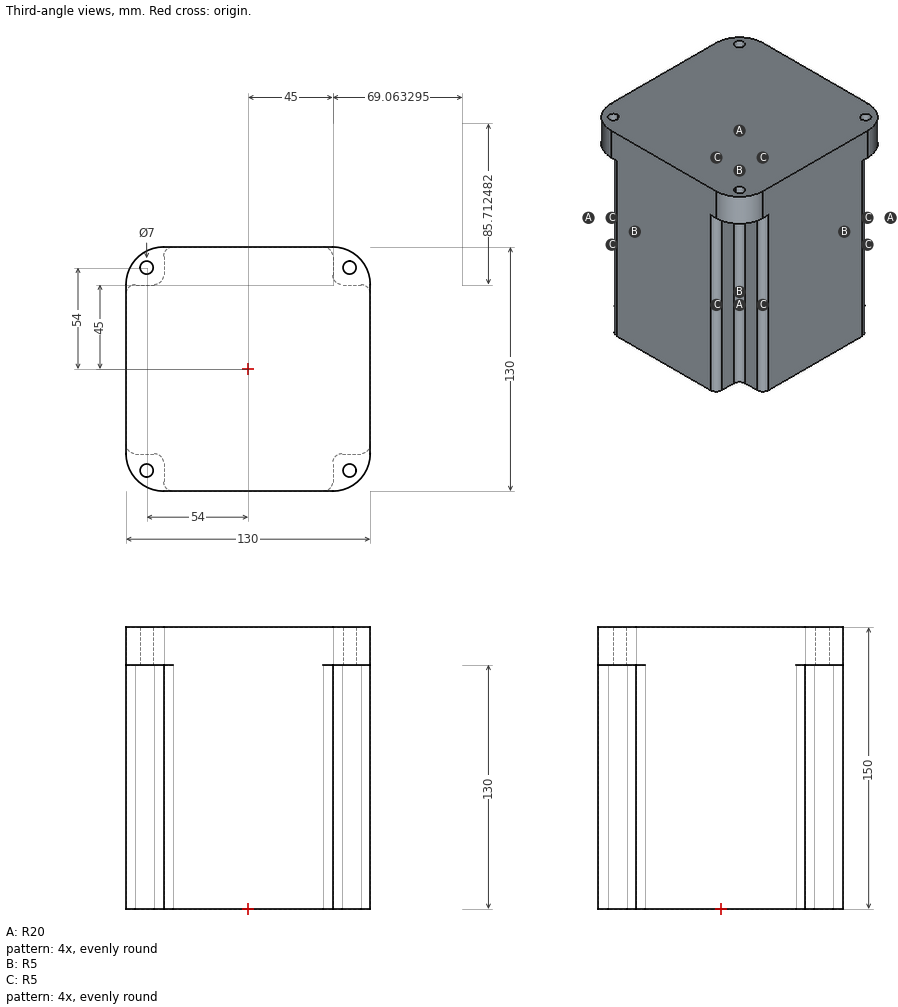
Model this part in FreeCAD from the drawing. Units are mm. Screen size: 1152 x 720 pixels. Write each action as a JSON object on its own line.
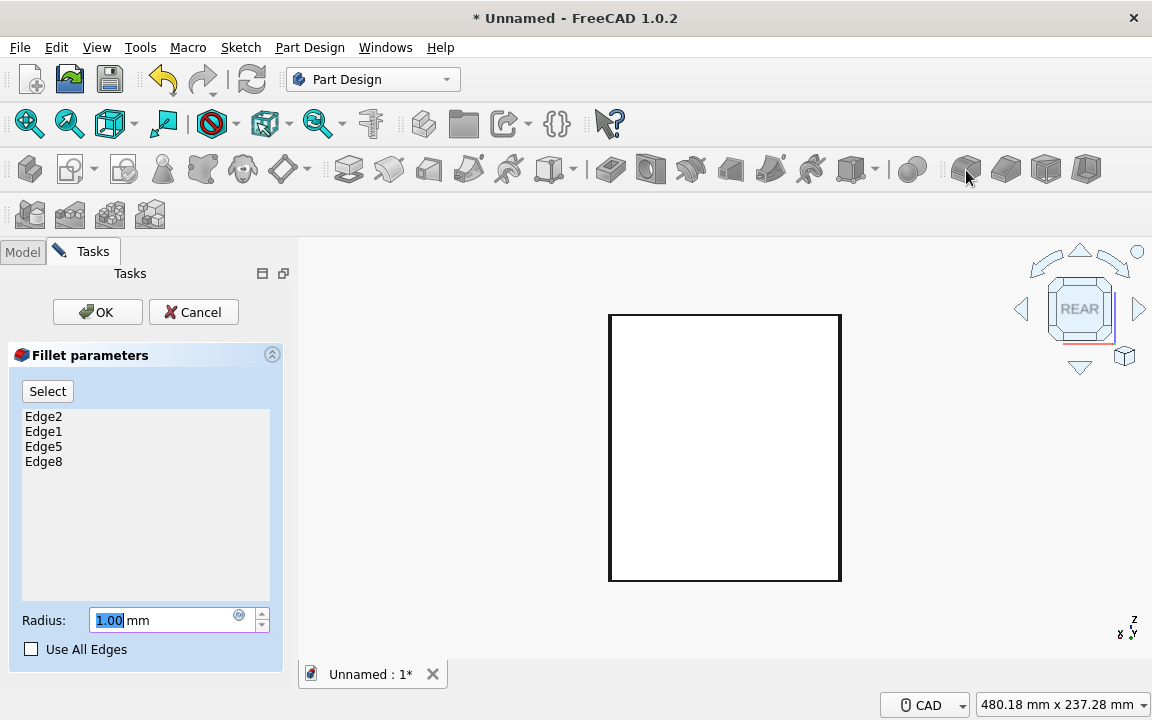
{"action": "type", "text": "20"}
{"action": "key", "text": "Tab"}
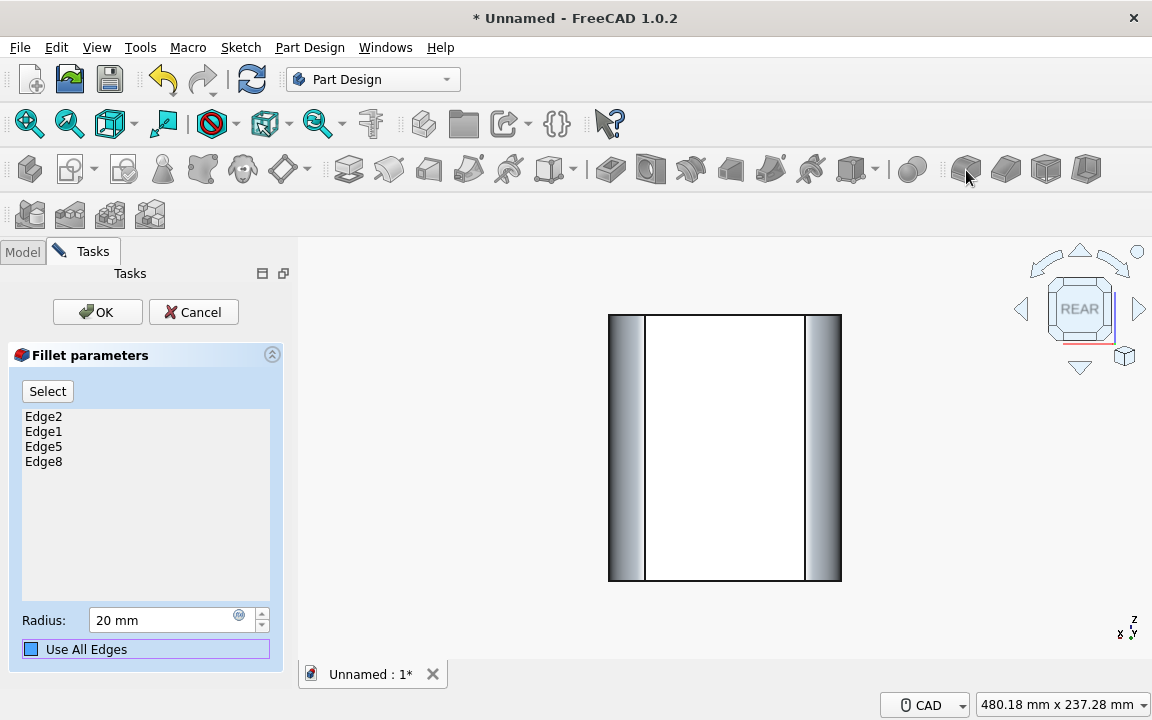
{"action": "left_click", "coordinate": [98, 312]}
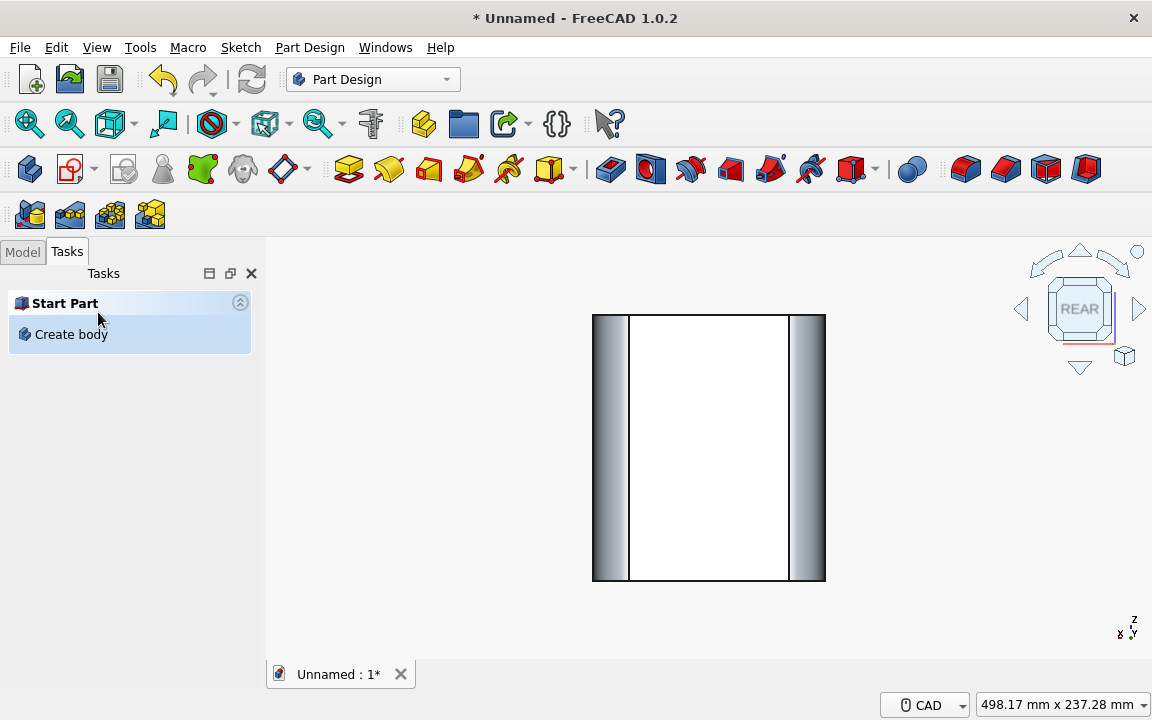
{"action": "left_click", "coordinate": [70, 170]}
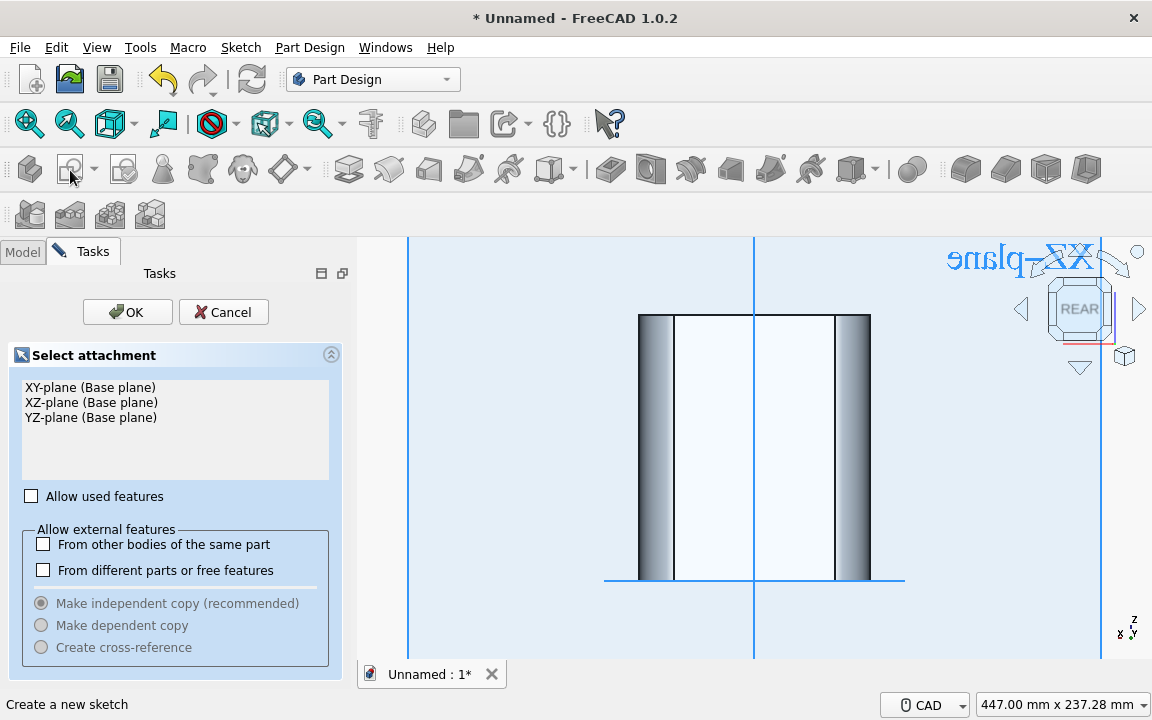
{"action": "left_click", "coordinate": [82, 388]}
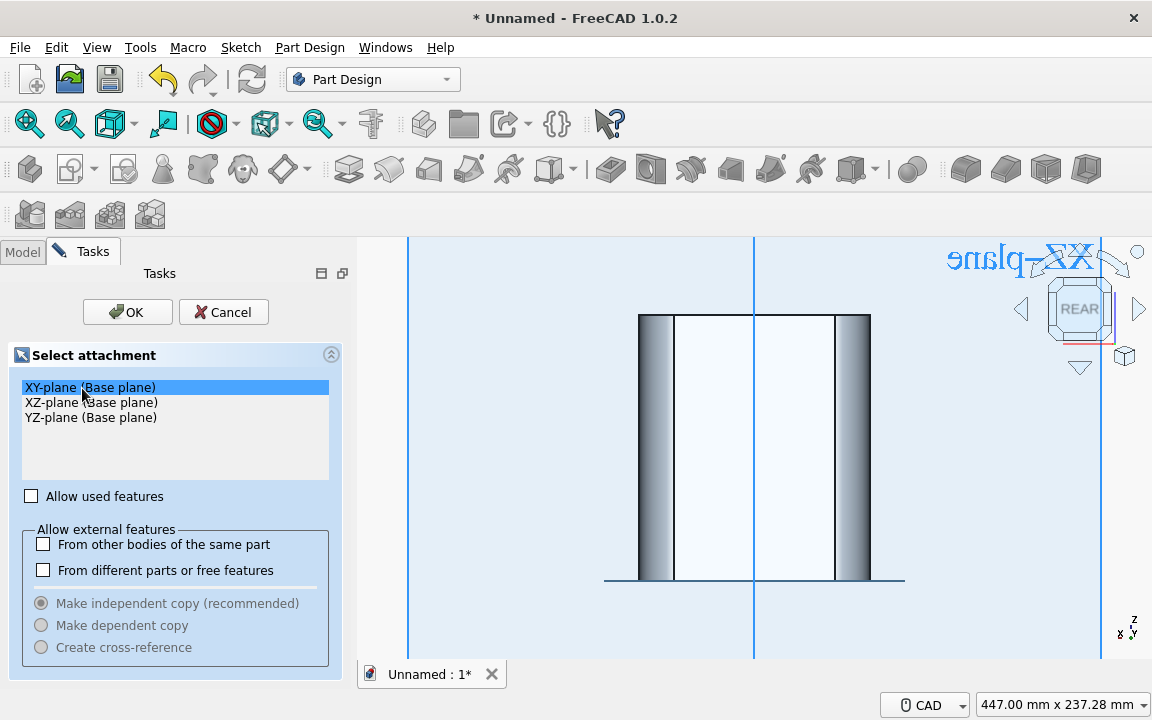
{"action": "left_click", "coordinate": [128, 312]}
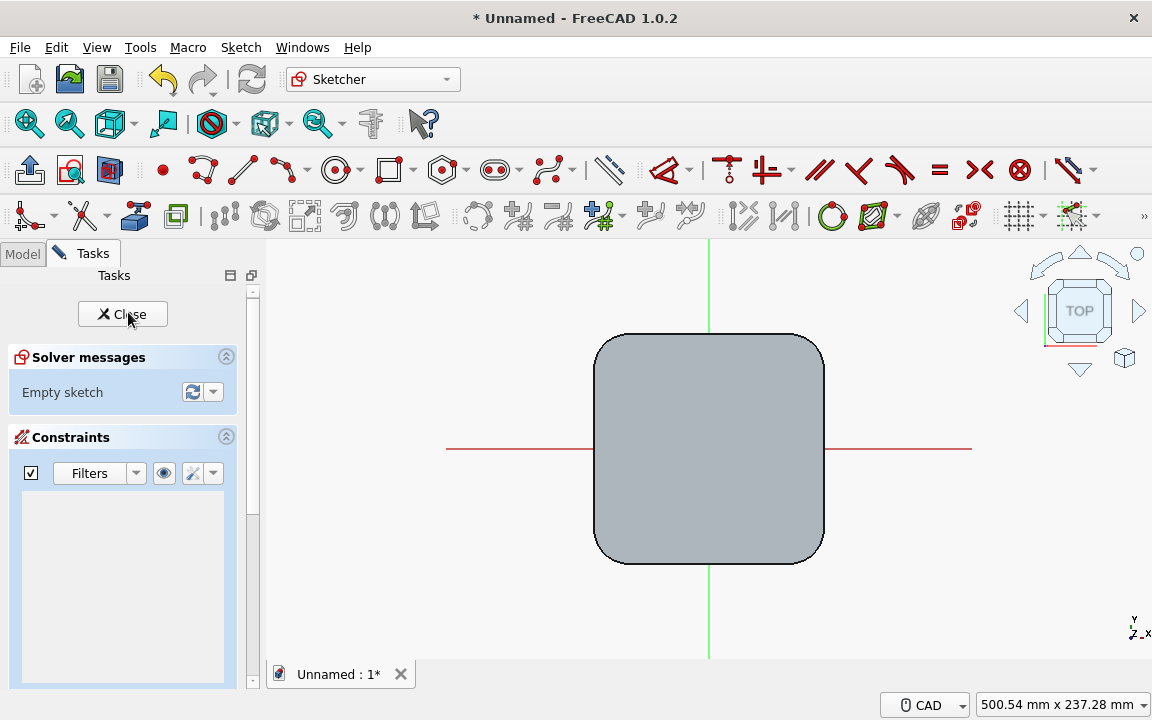
{"action": "key", "text": "q s"}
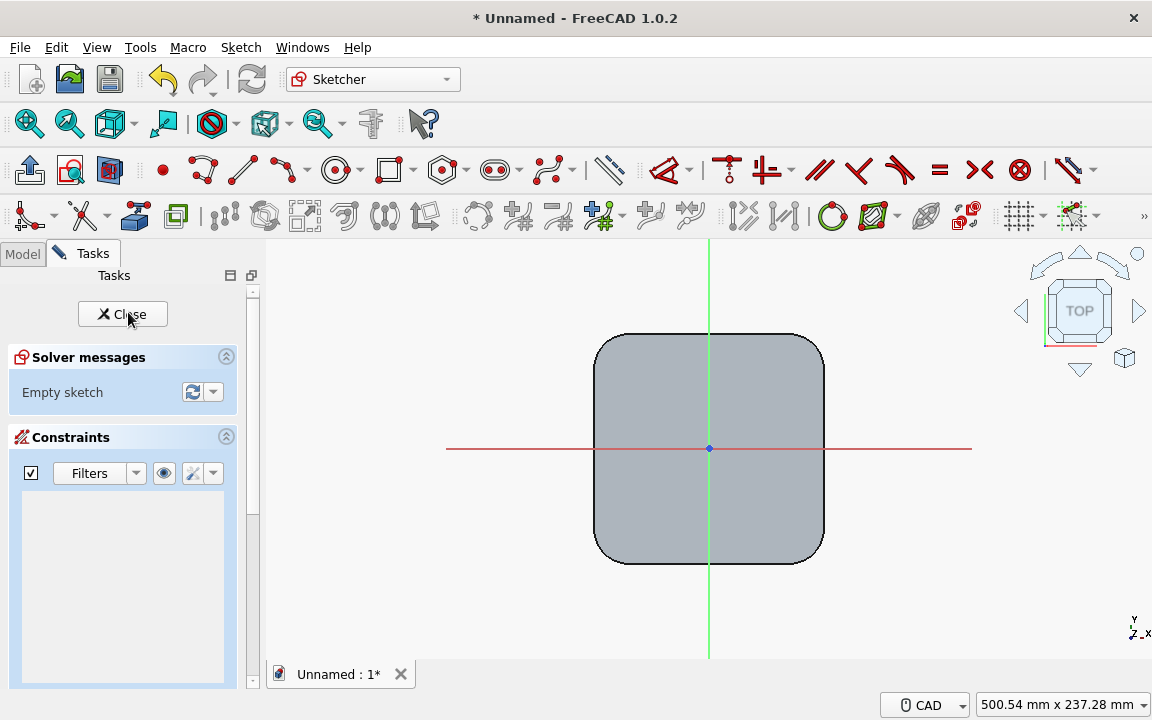
{"action": "scroll", "coordinate": [294, 631], "scroll_direction": "down", "scroll_amount": 1}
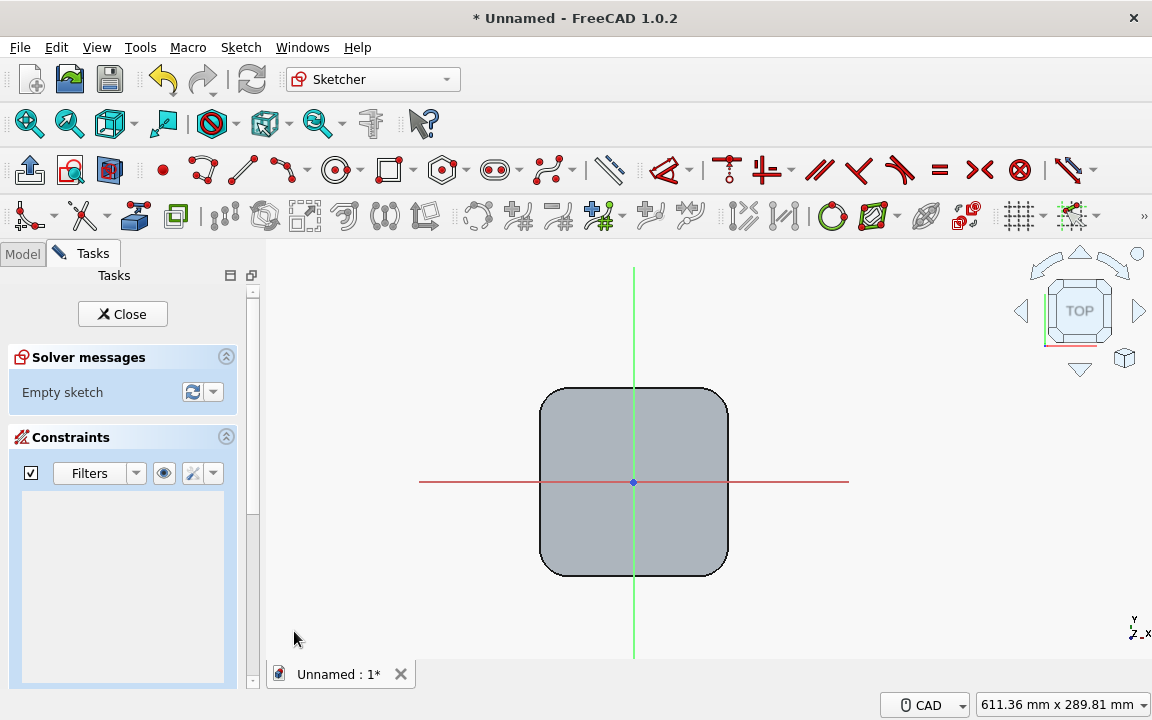
{"action": "scroll", "coordinate": [871, 267], "scroll_direction": "up", "scroll_amount": 2}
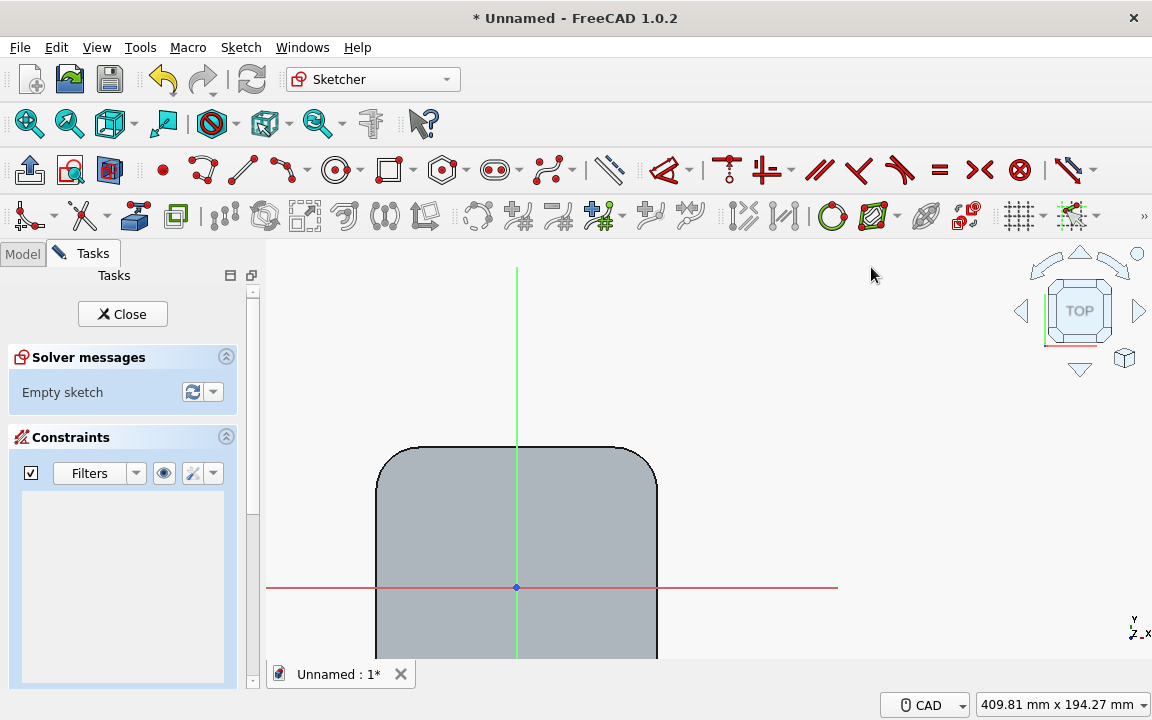
{"action": "left_click", "coordinate": [390, 170]}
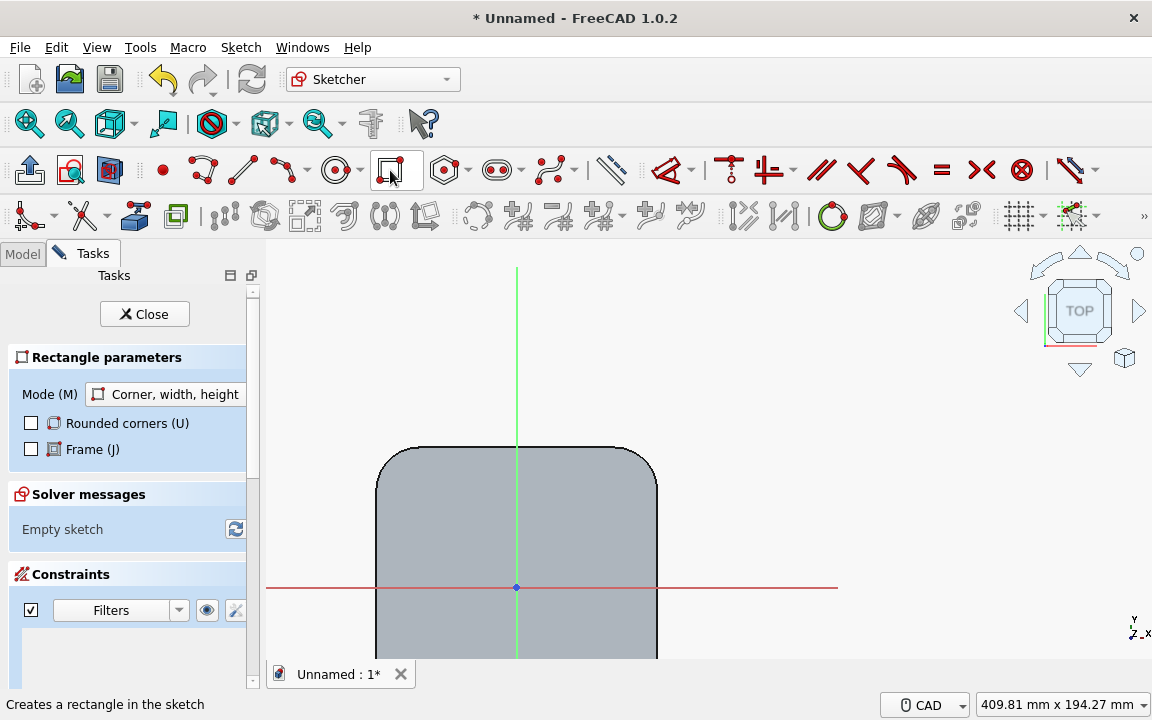
{"action": "left_click", "coordinate": [614, 305]}
{"action": "mouse_move", "coordinate": [763, 491]}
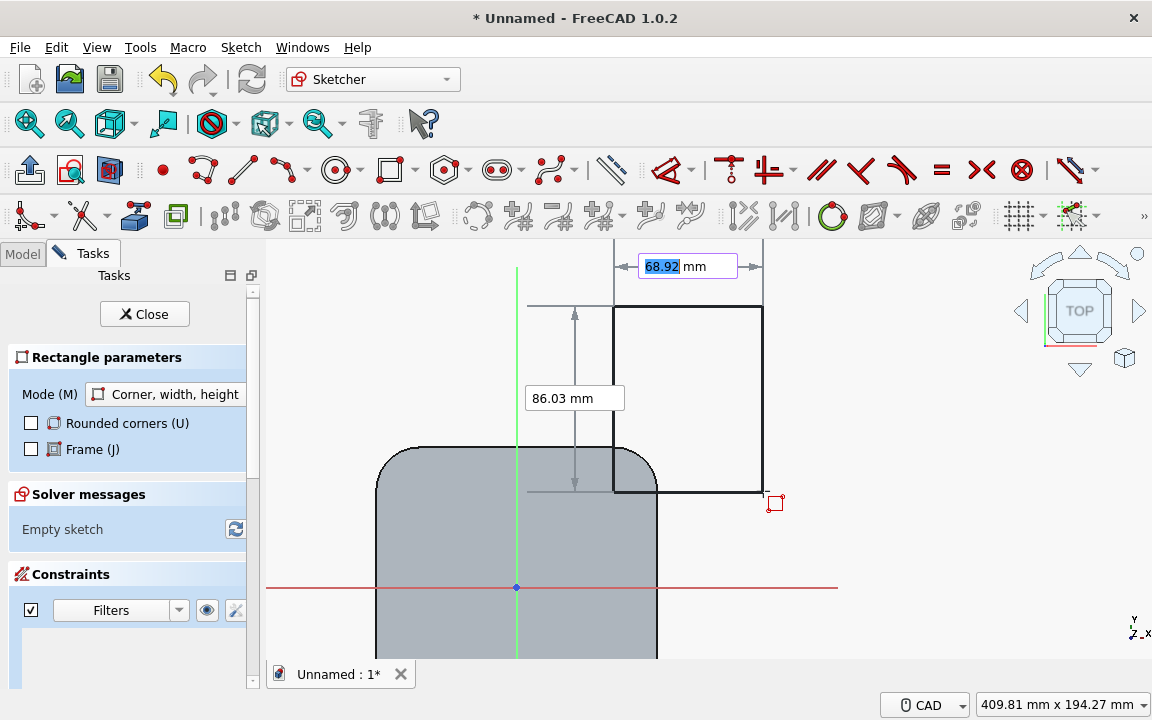
{"action": "type", "text": "69.063295"}
{"action": "key", "text": "Tab"}
{"action": "type", "text": "85.712482"}
{"action": "key", "text": "Return"}
{"action": "key", "text": "Escape"}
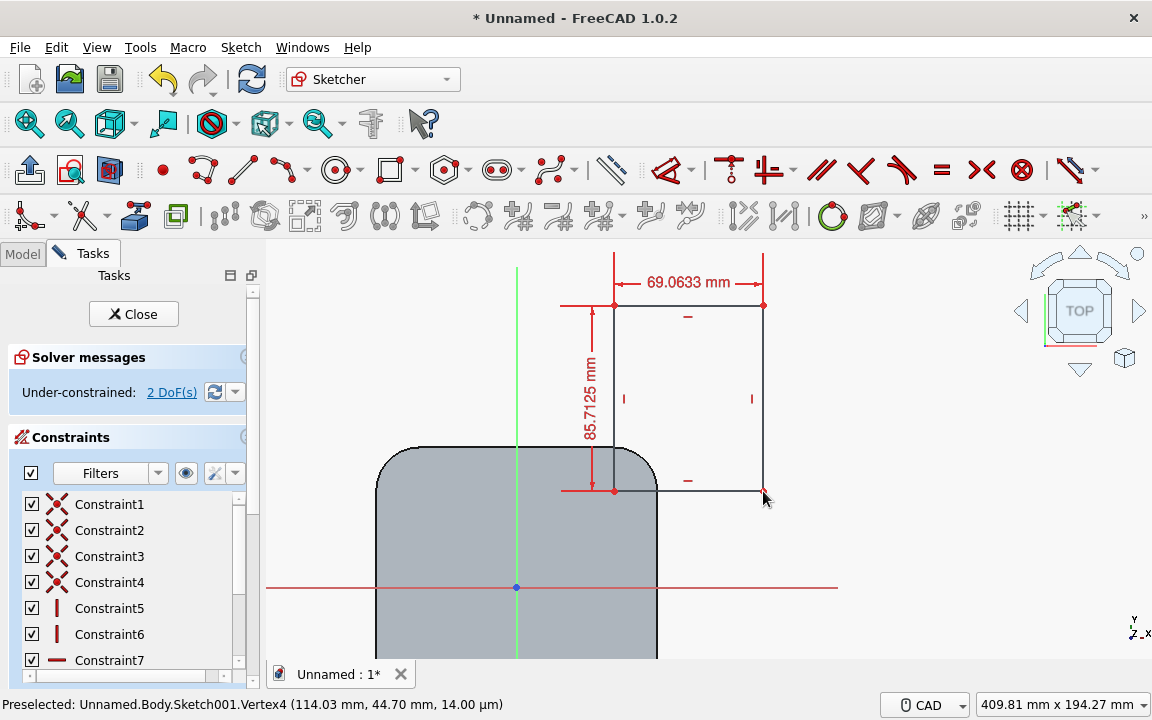
{"action": "key", "text": "d"}